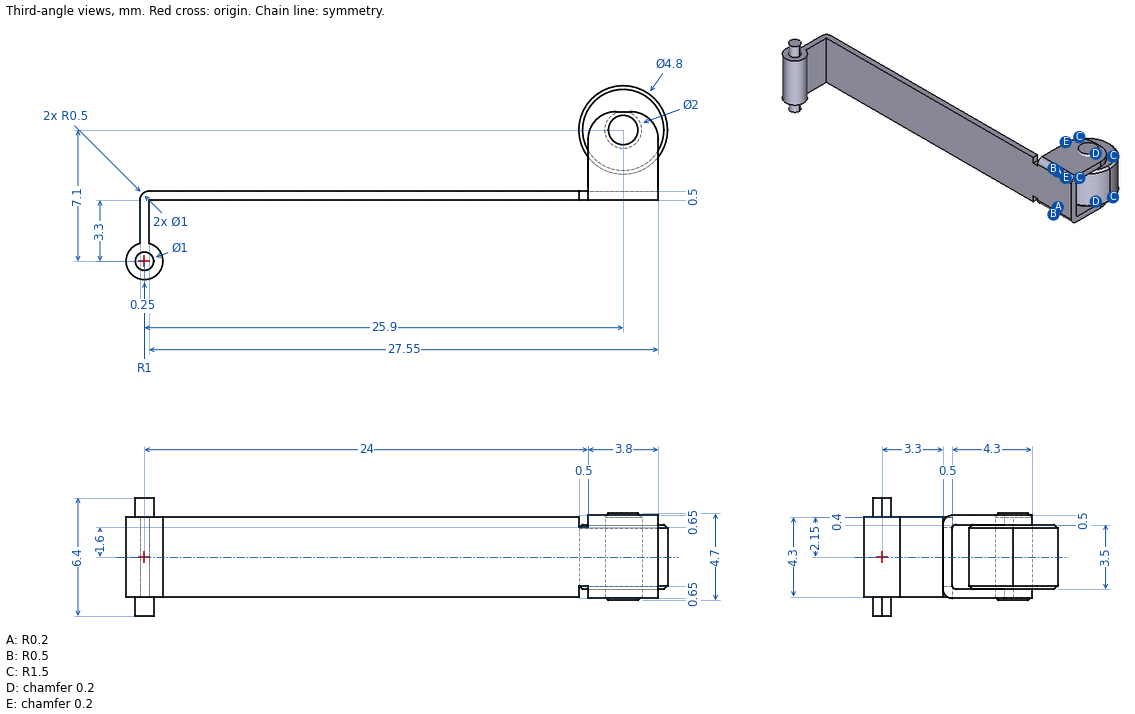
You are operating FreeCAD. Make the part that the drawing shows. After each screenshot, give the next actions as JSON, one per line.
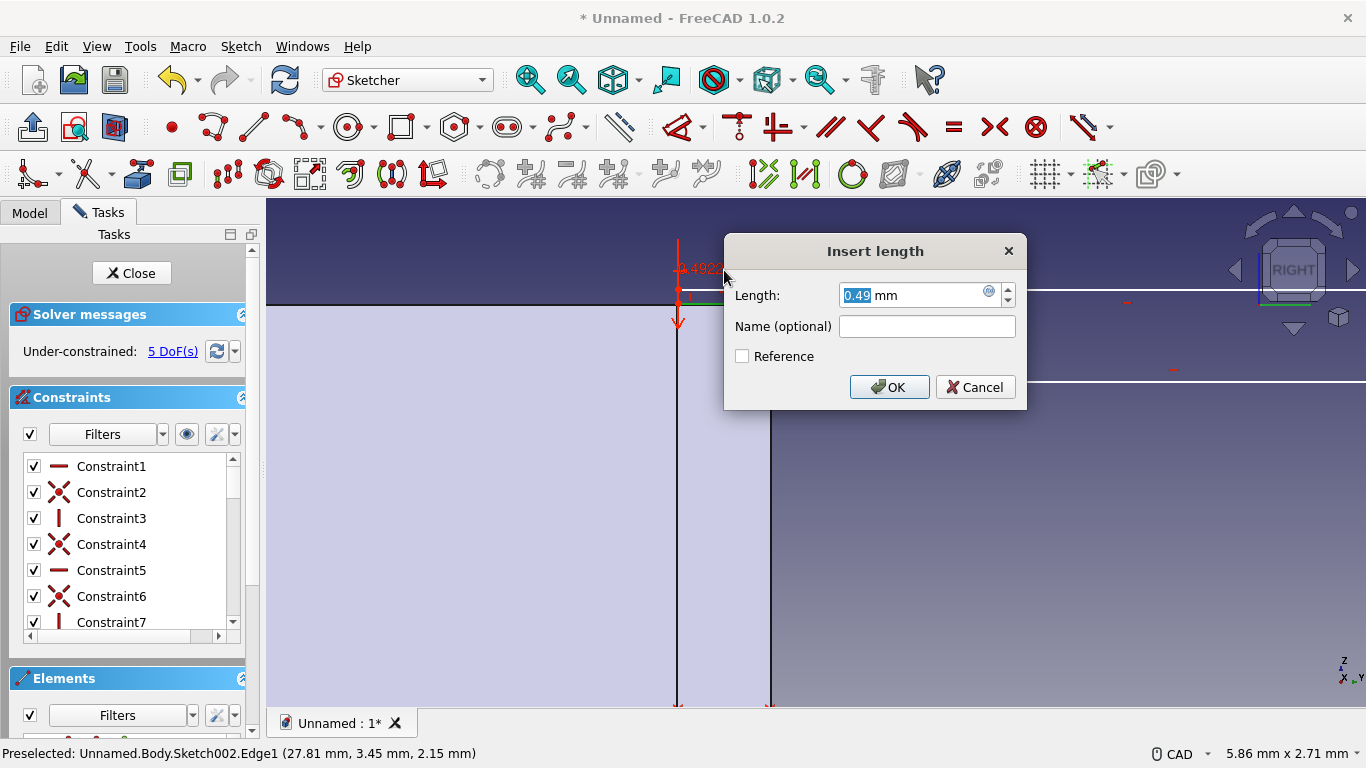
{"action": "type", "text": "0.5"}
{"action": "key", "text": "Return"}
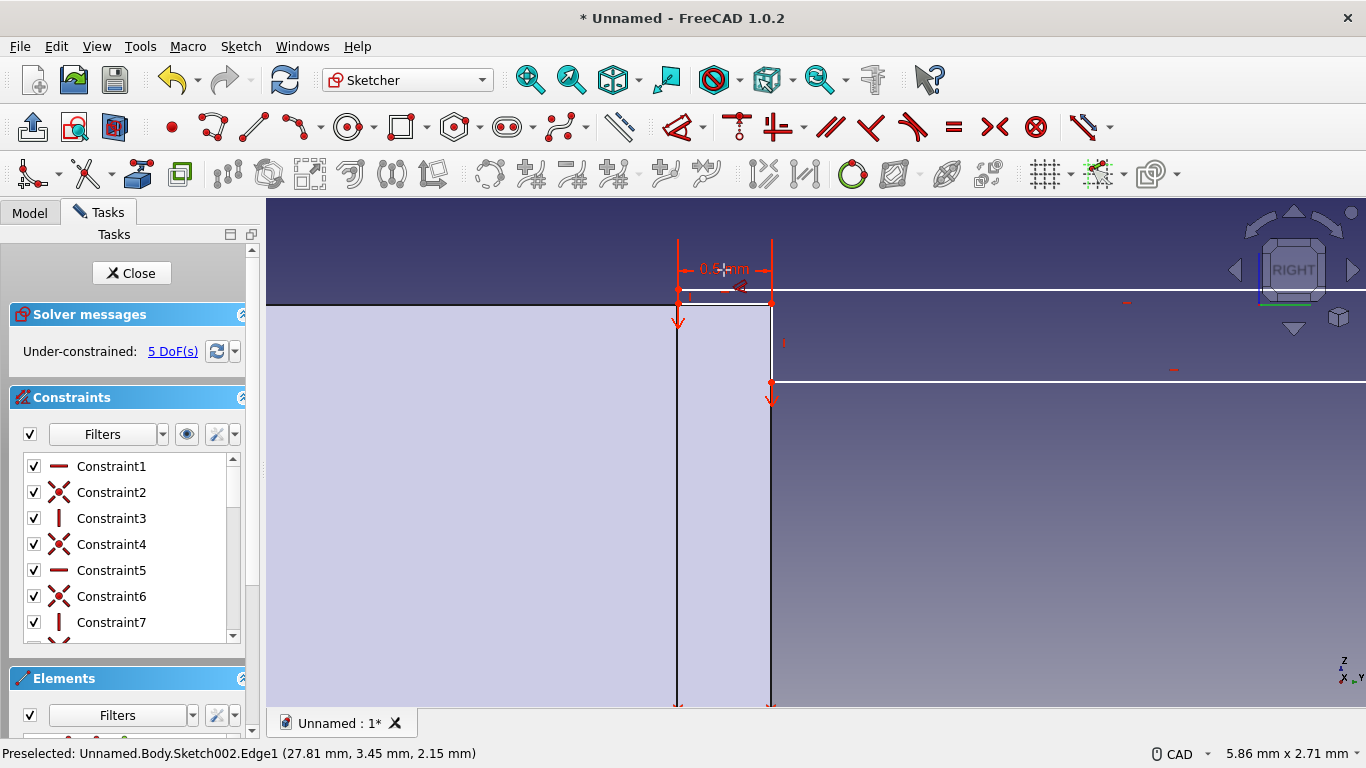
{"action": "left_click", "coordinate": [772, 327]}
{"action": "left_click", "coordinate": [738, 343]}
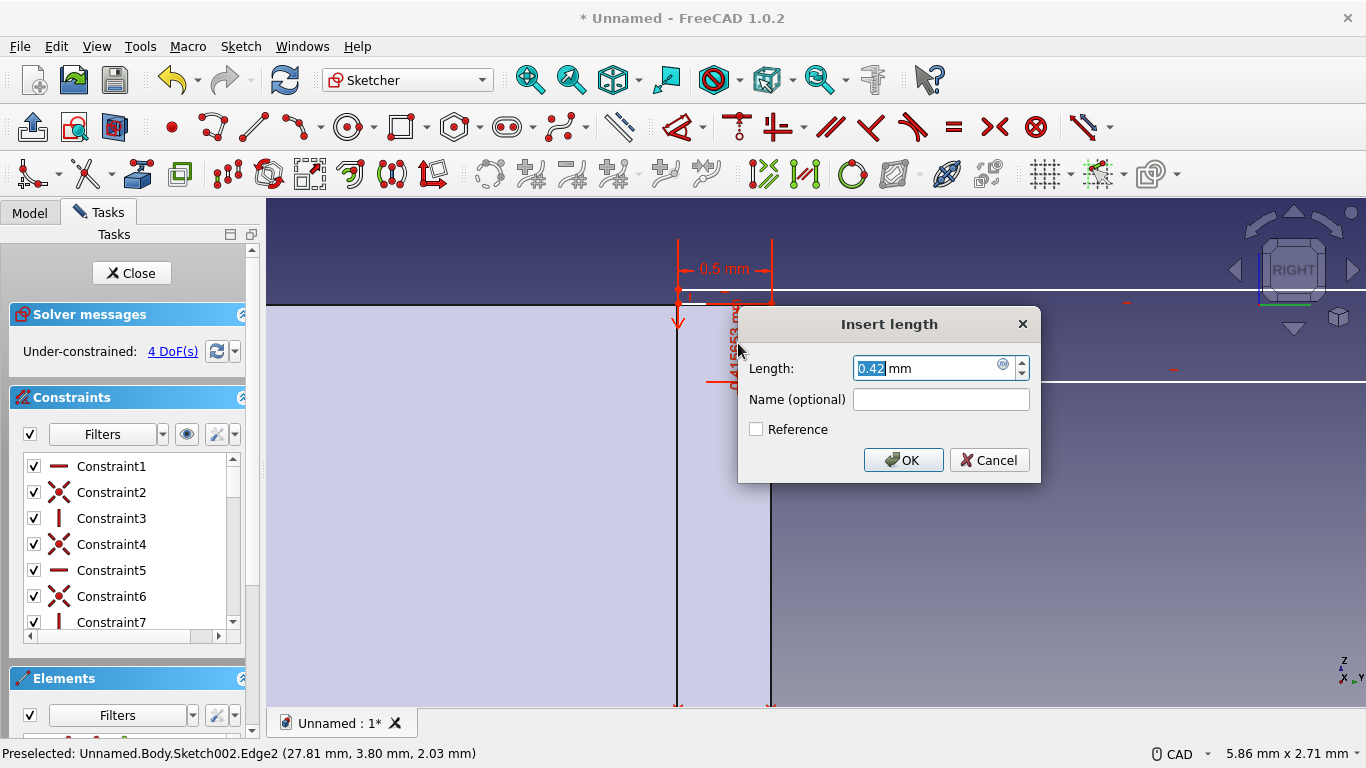
{"action": "type", "text": "0.4"}
{"action": "key", "text": "Return"}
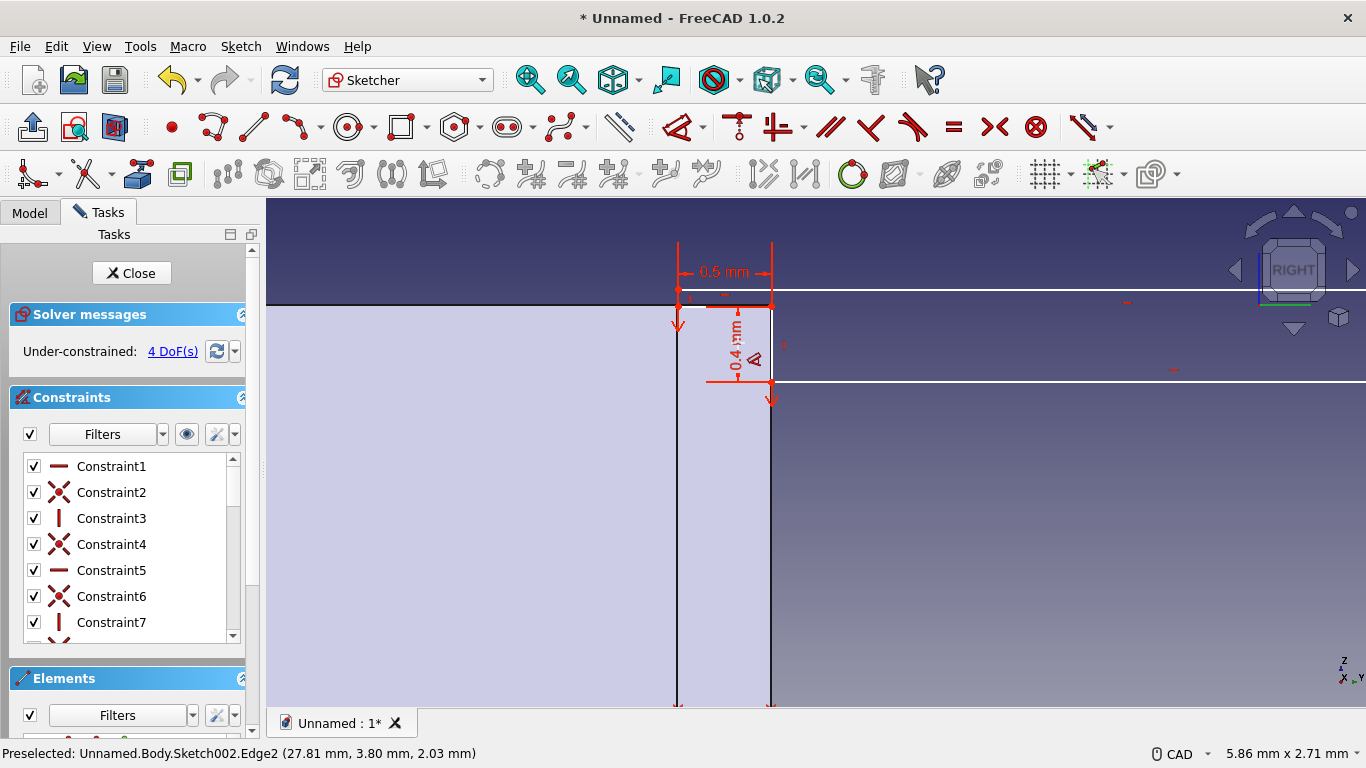
{"action": "left_click", "coordinate": [1014, 382]}
{"action": "left_click", "coordinate": [986, 348]}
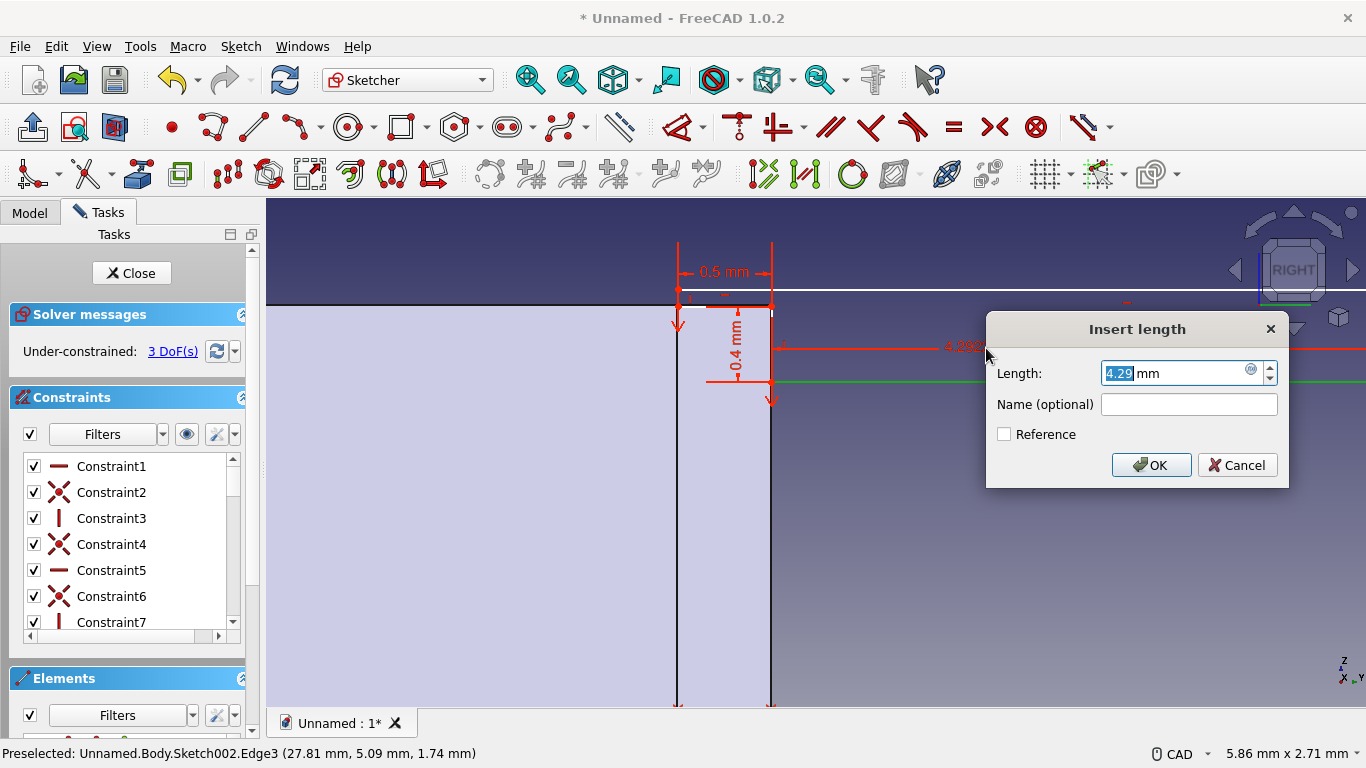
{"action": "type", "text": "4.3"}
{"action": "key", "text": "Return"}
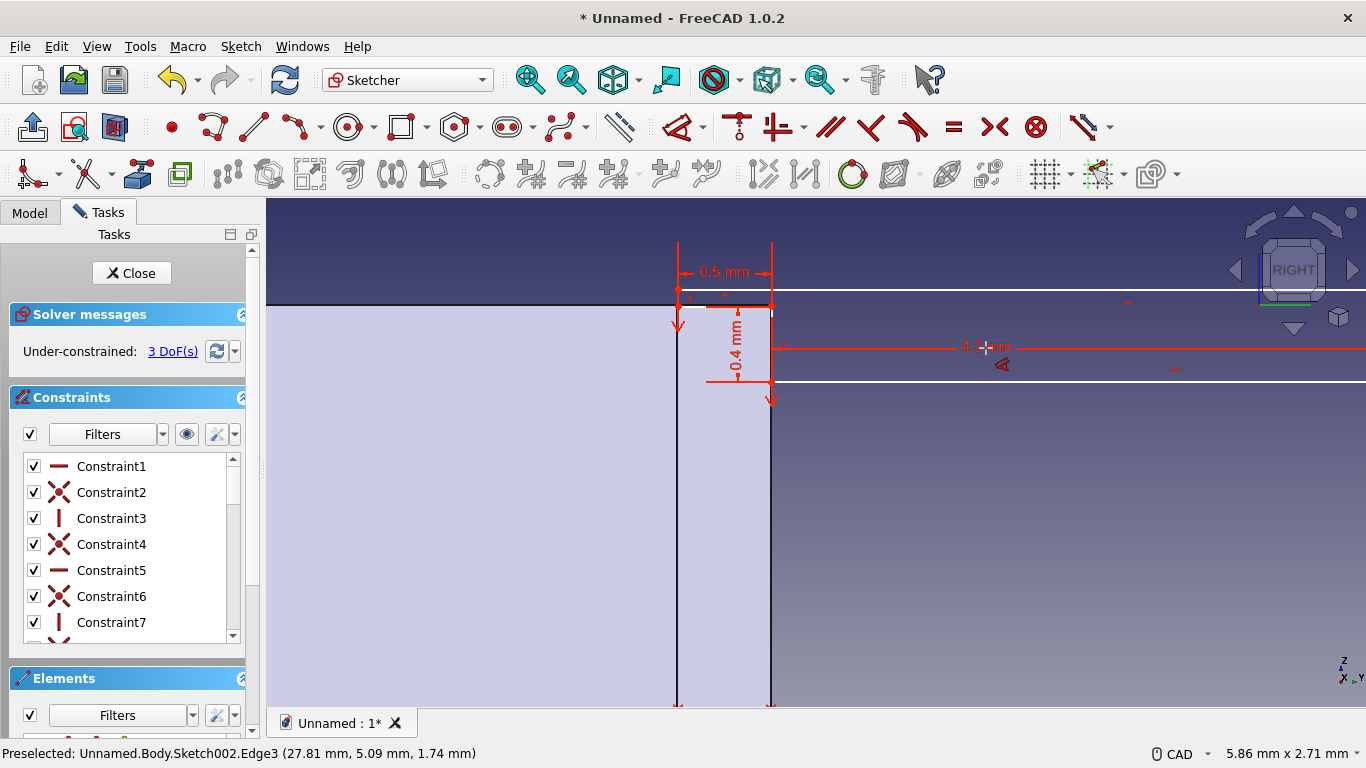
{"action": "scroll", "coordinate": [706, 304], "scroll_direction": "down", "scroll_amount": 5}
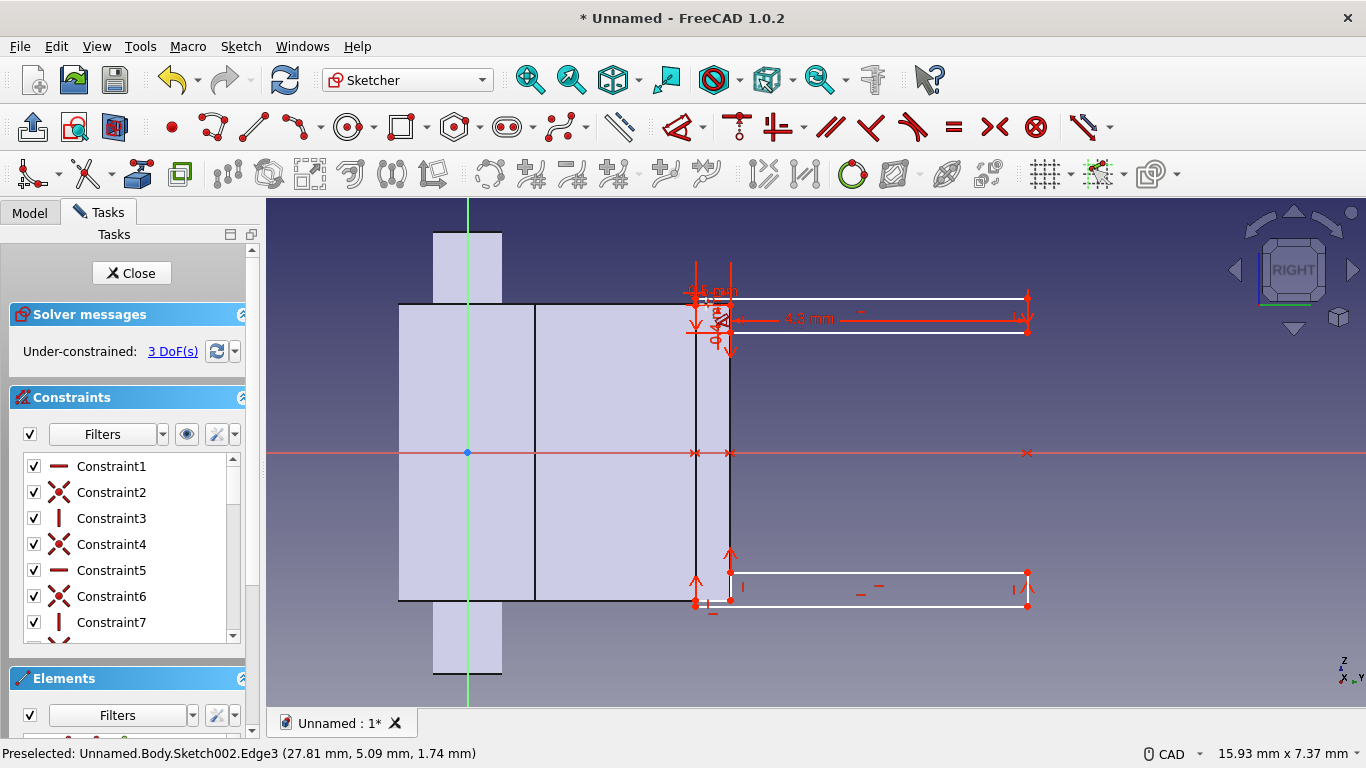
{"action": "scroll", "coordinate": [1028, 323], "scroll_direction": "up", "scroll_amount": 2}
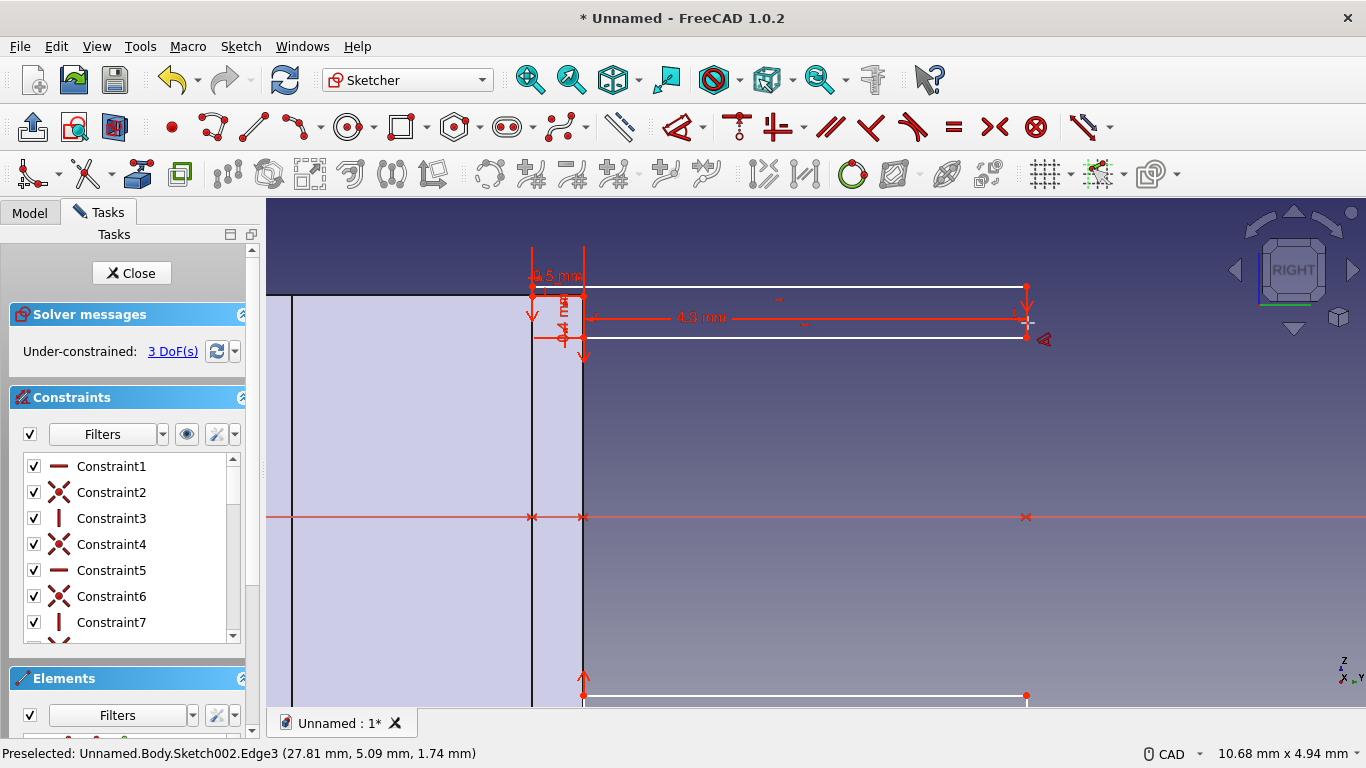
{"action": "left_click", "coordinate": [1027, 322]}
{"action": "left_click", "coordinate": [1061, 312]}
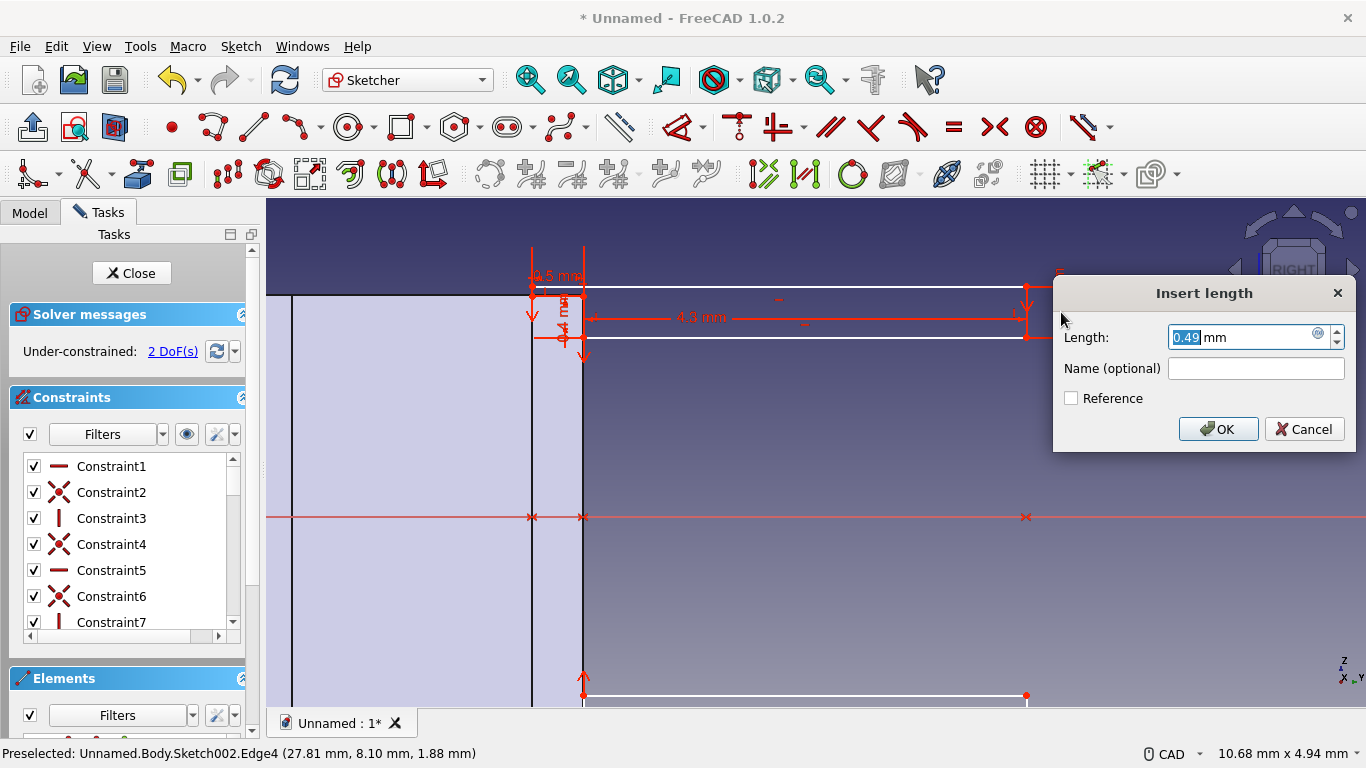
{"action": "type", "text": "0.5"}
{"action": "key", "text": "Return"}